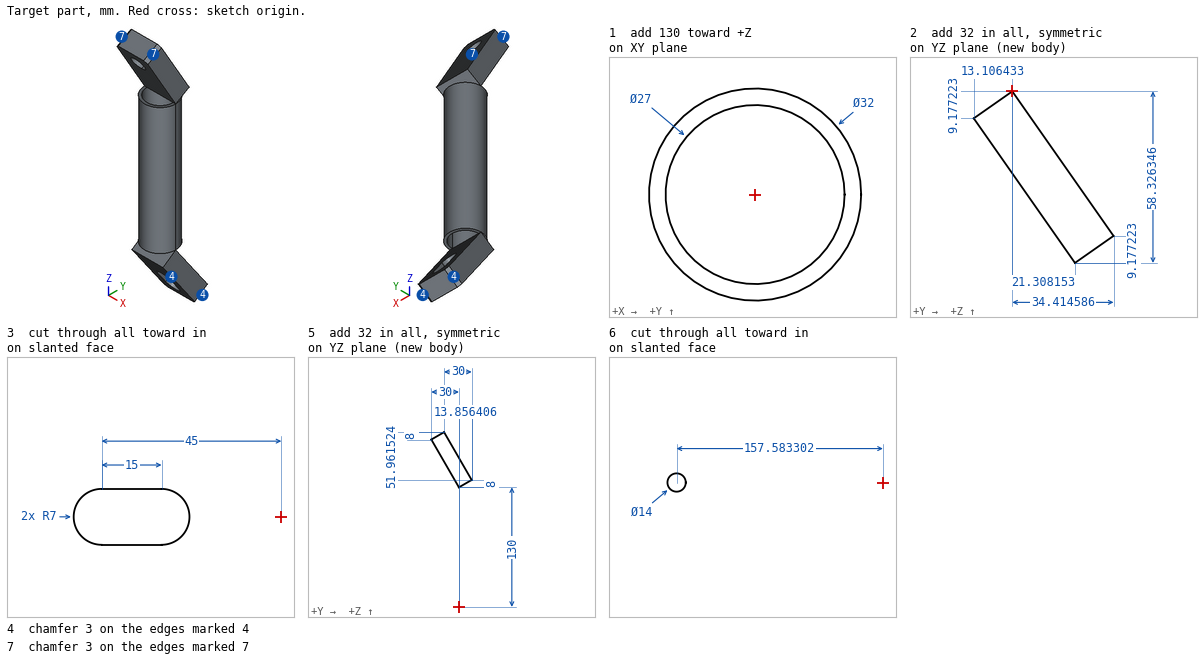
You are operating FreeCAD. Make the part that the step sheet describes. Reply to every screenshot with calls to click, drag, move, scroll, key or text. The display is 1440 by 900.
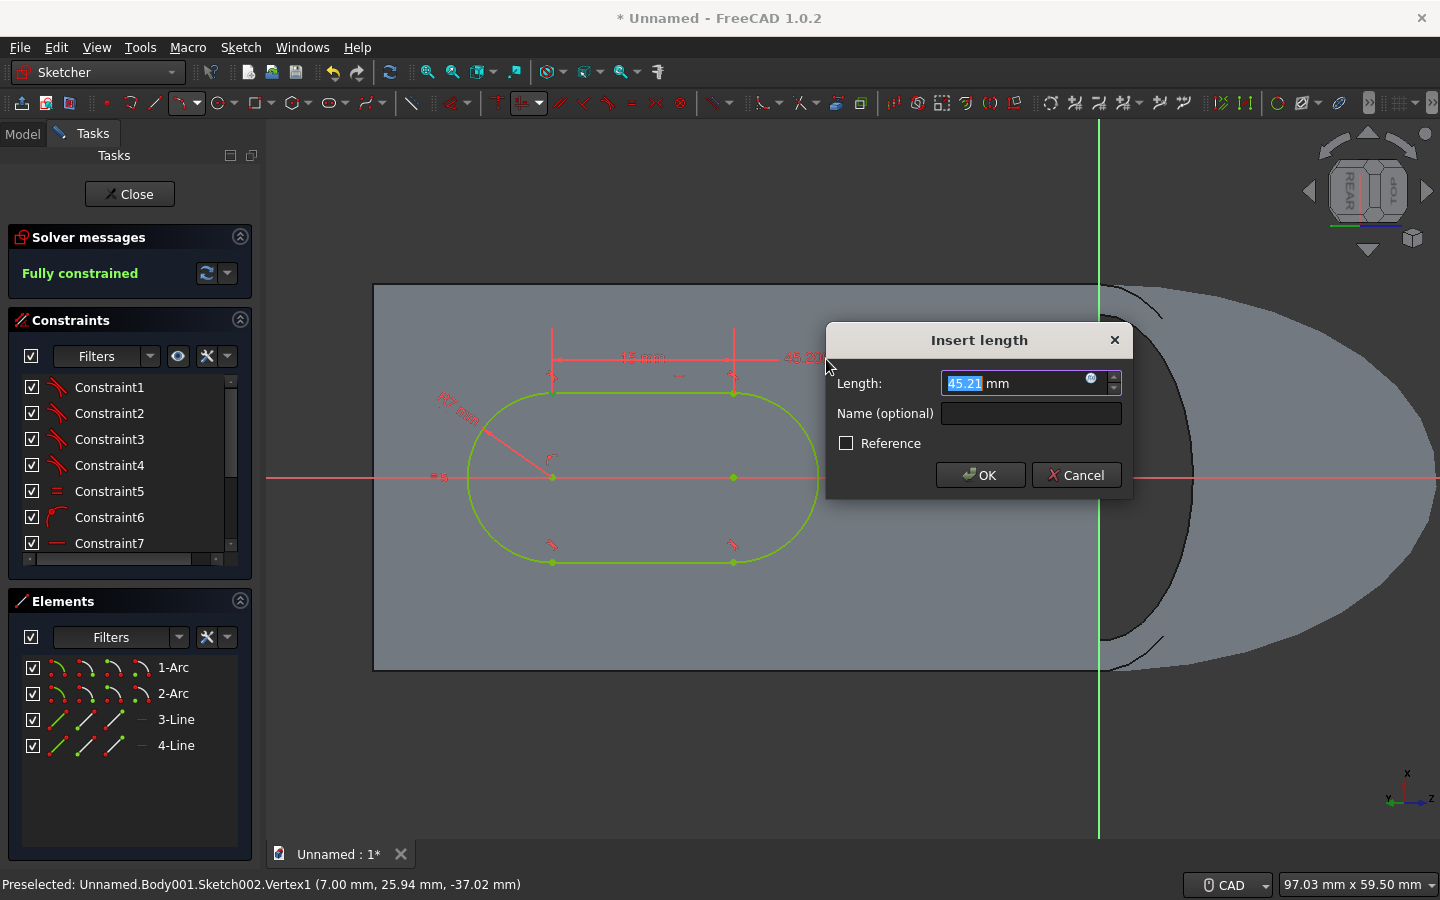
text(45)
key(Return)
key(Escape)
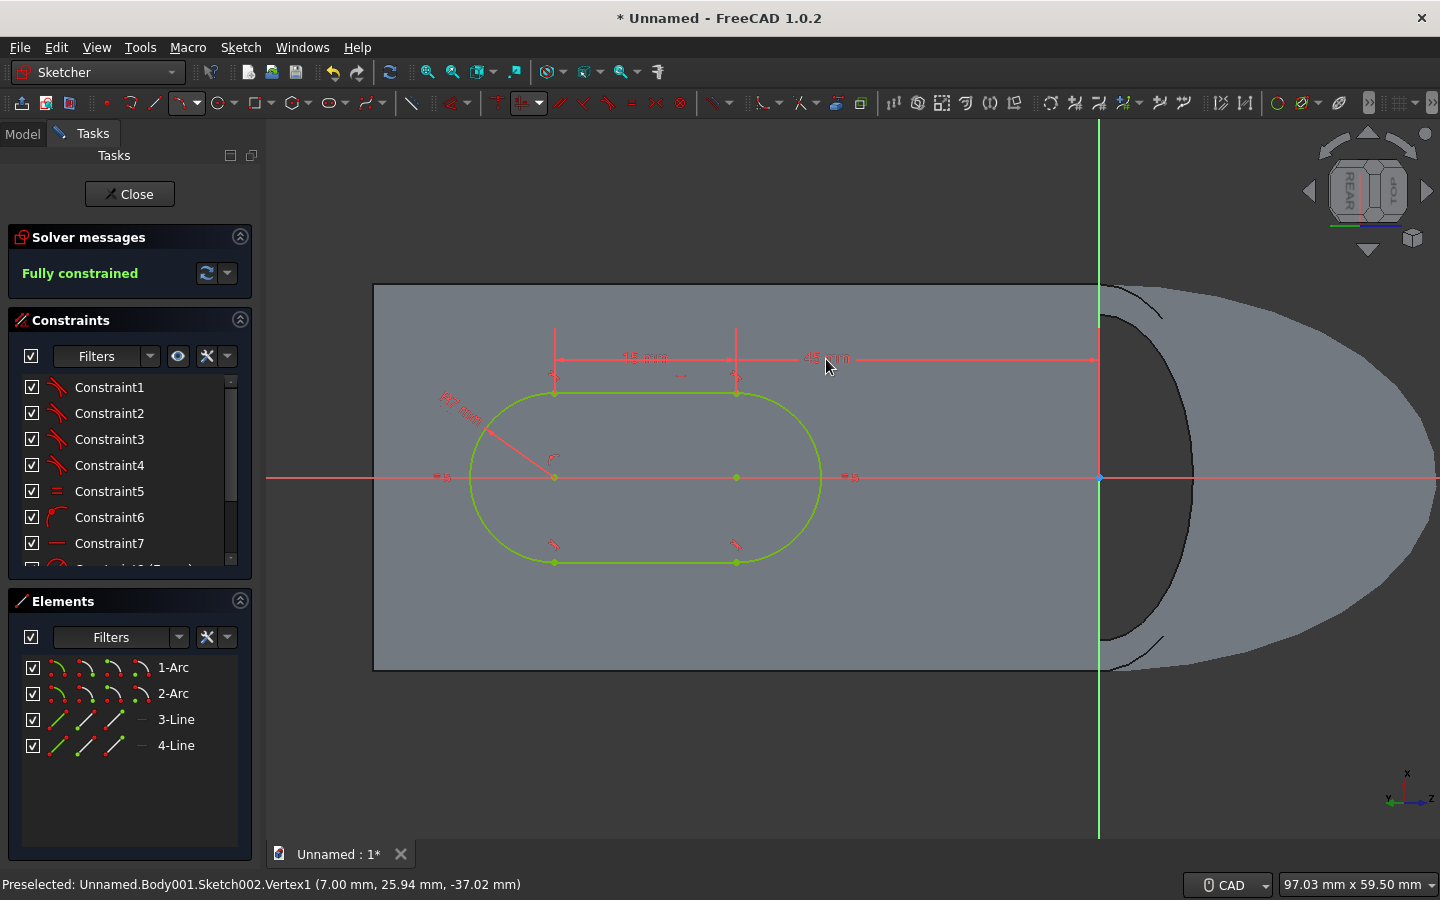
click(130, 194)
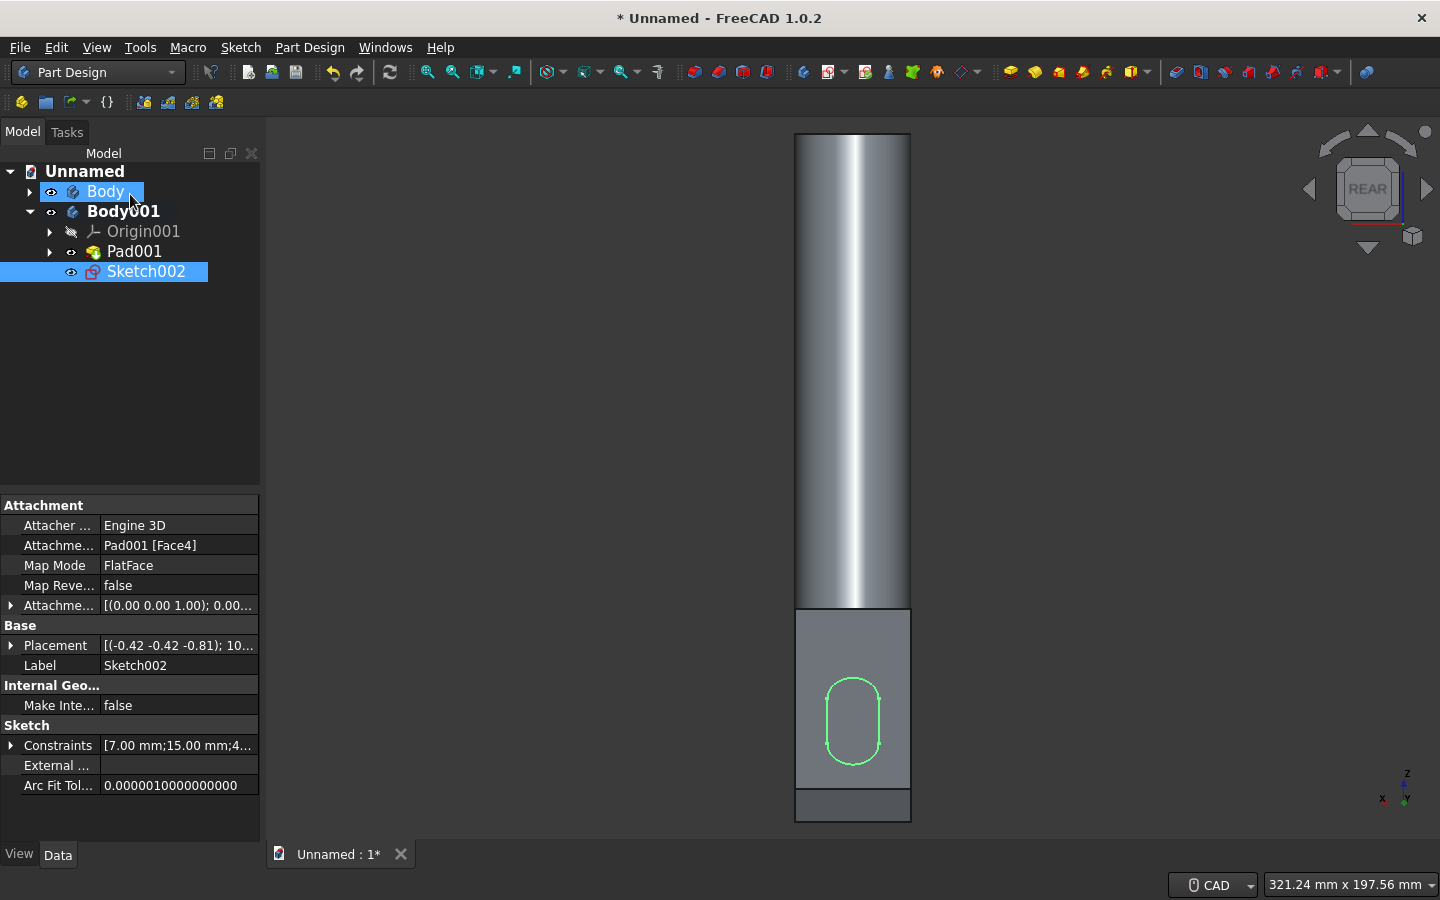
click(1178, 72)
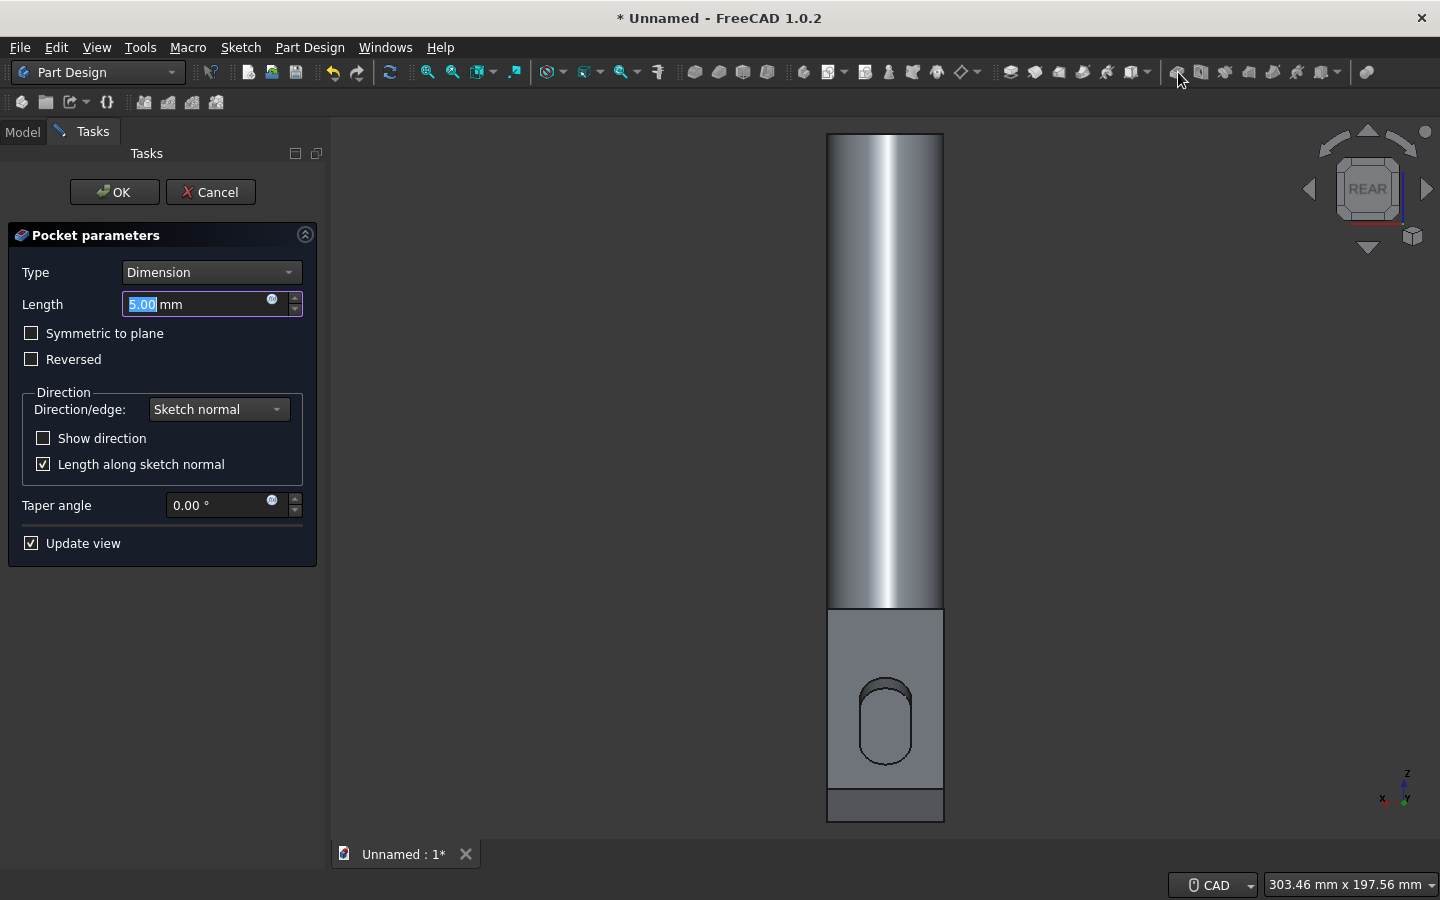
click(212, 272)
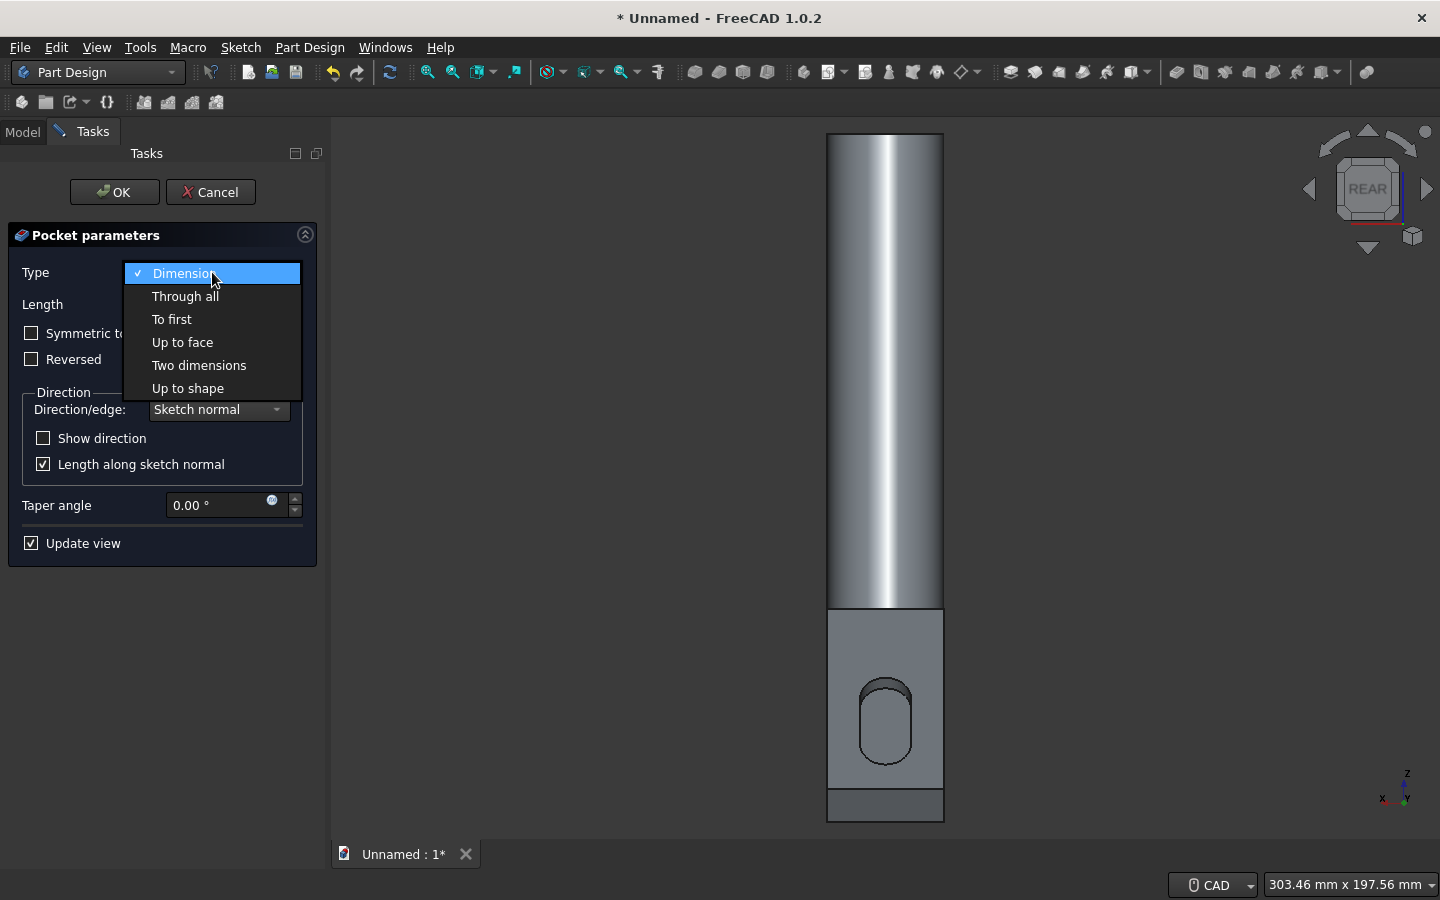
click(212, 296)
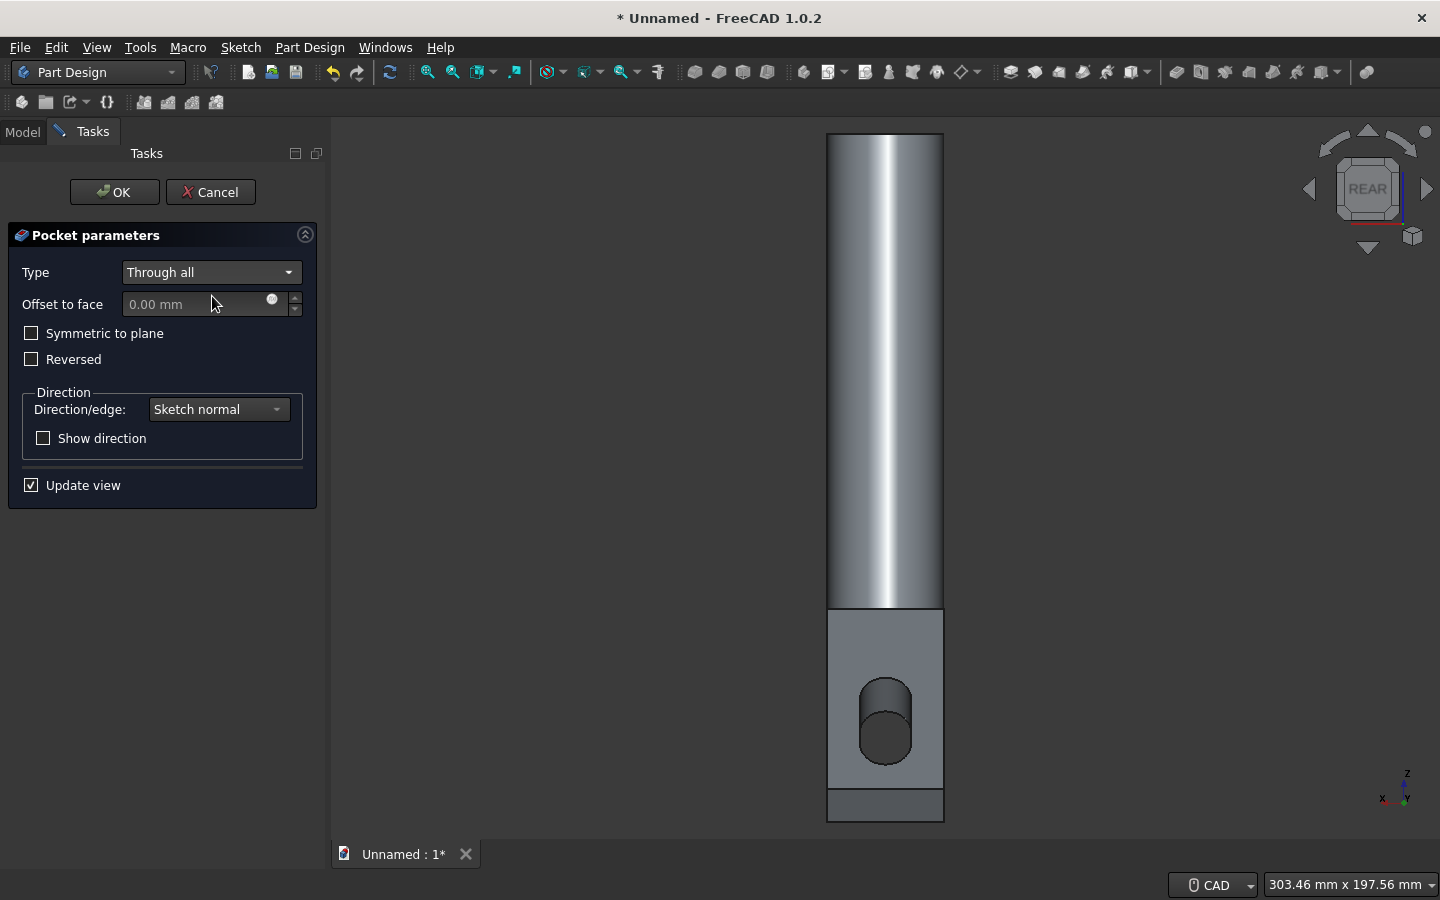
click(115, 192)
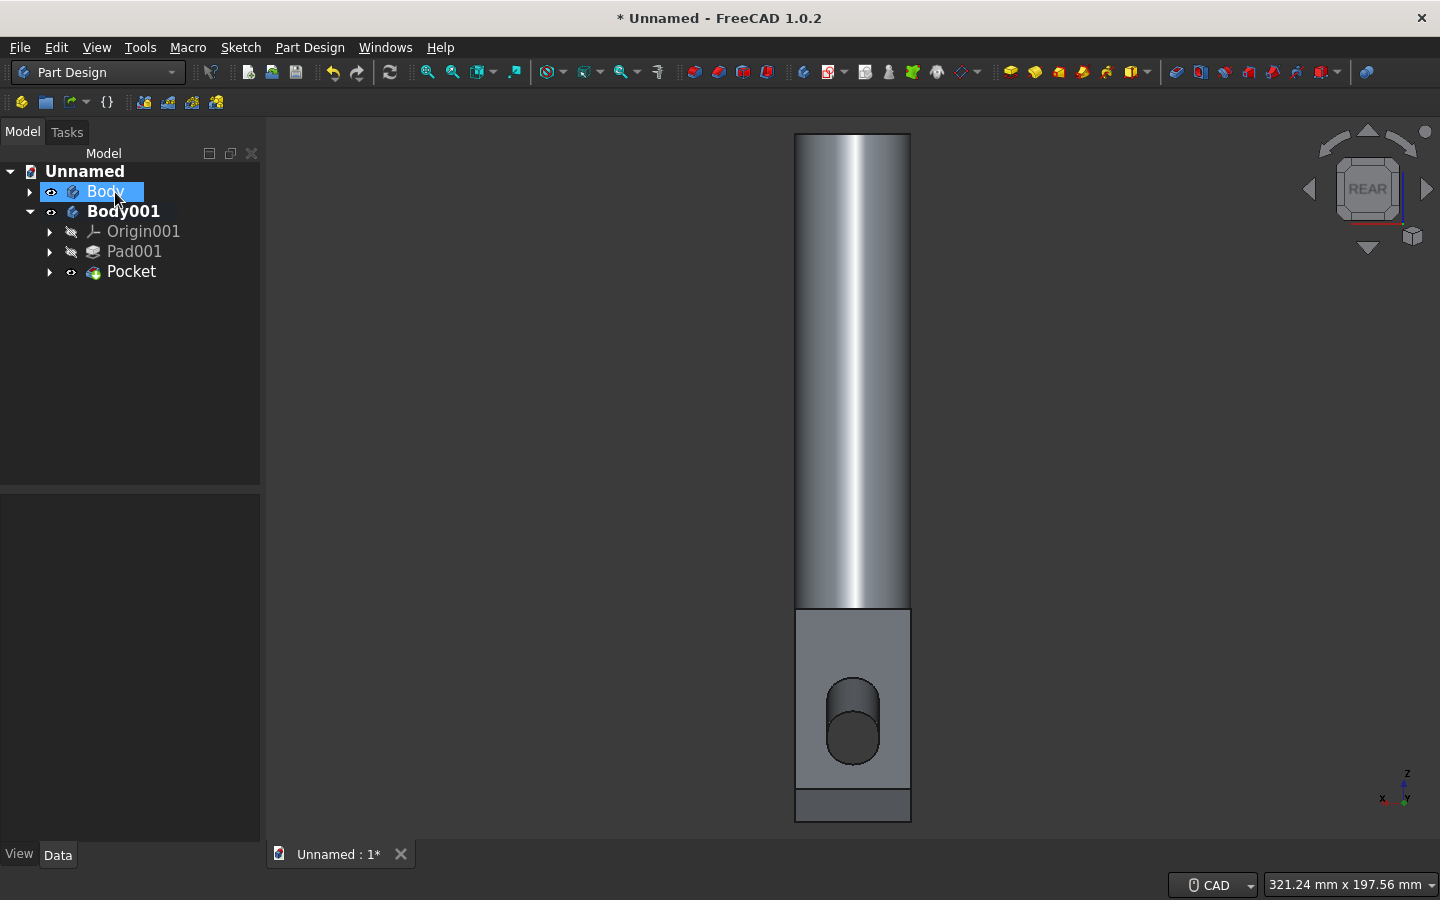
key(v)
key(f)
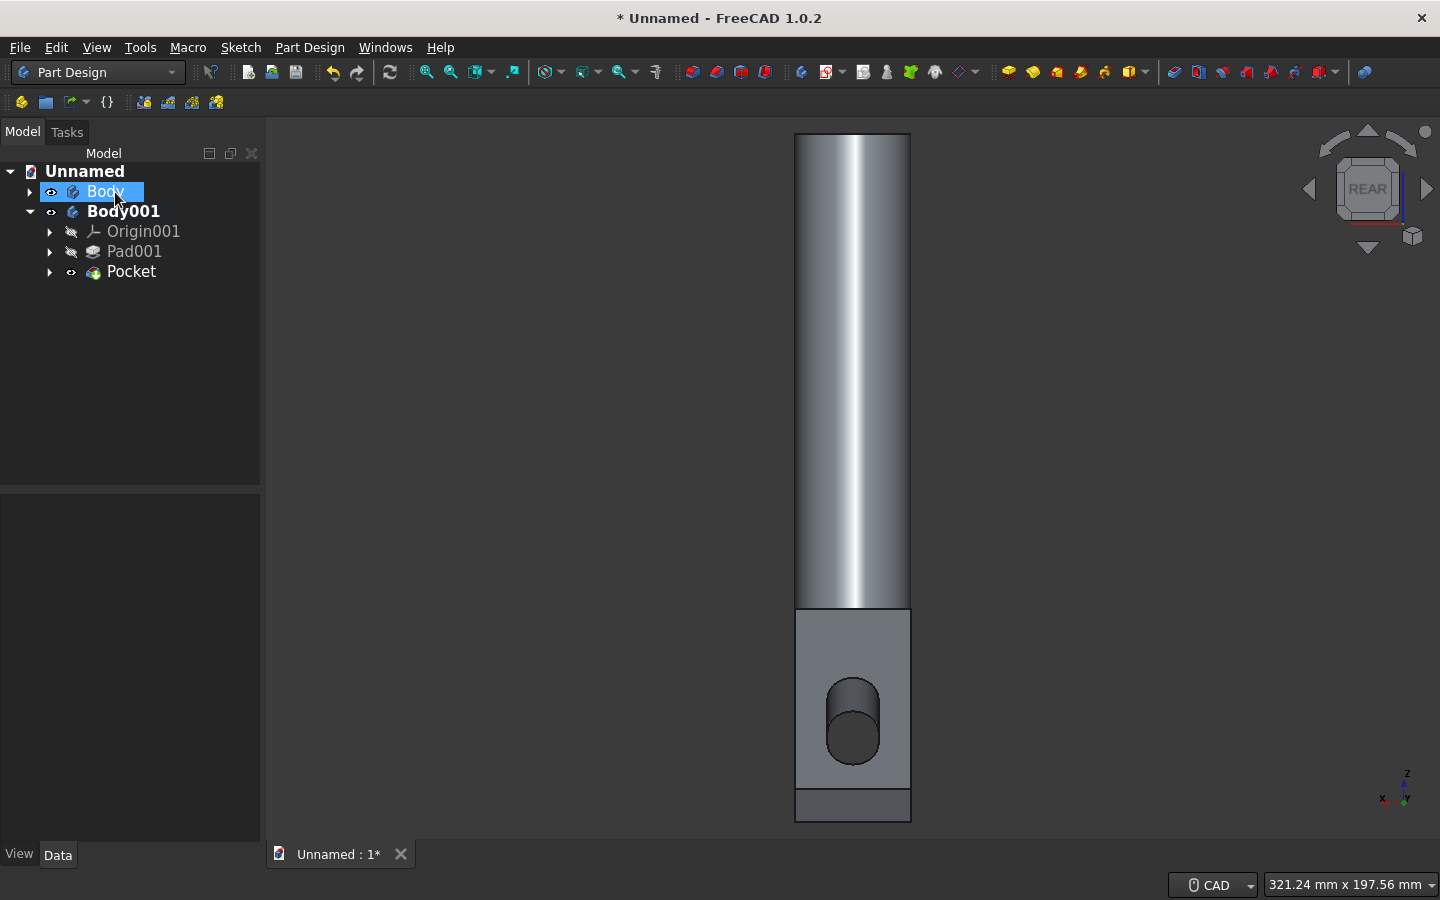
click(911, 804)